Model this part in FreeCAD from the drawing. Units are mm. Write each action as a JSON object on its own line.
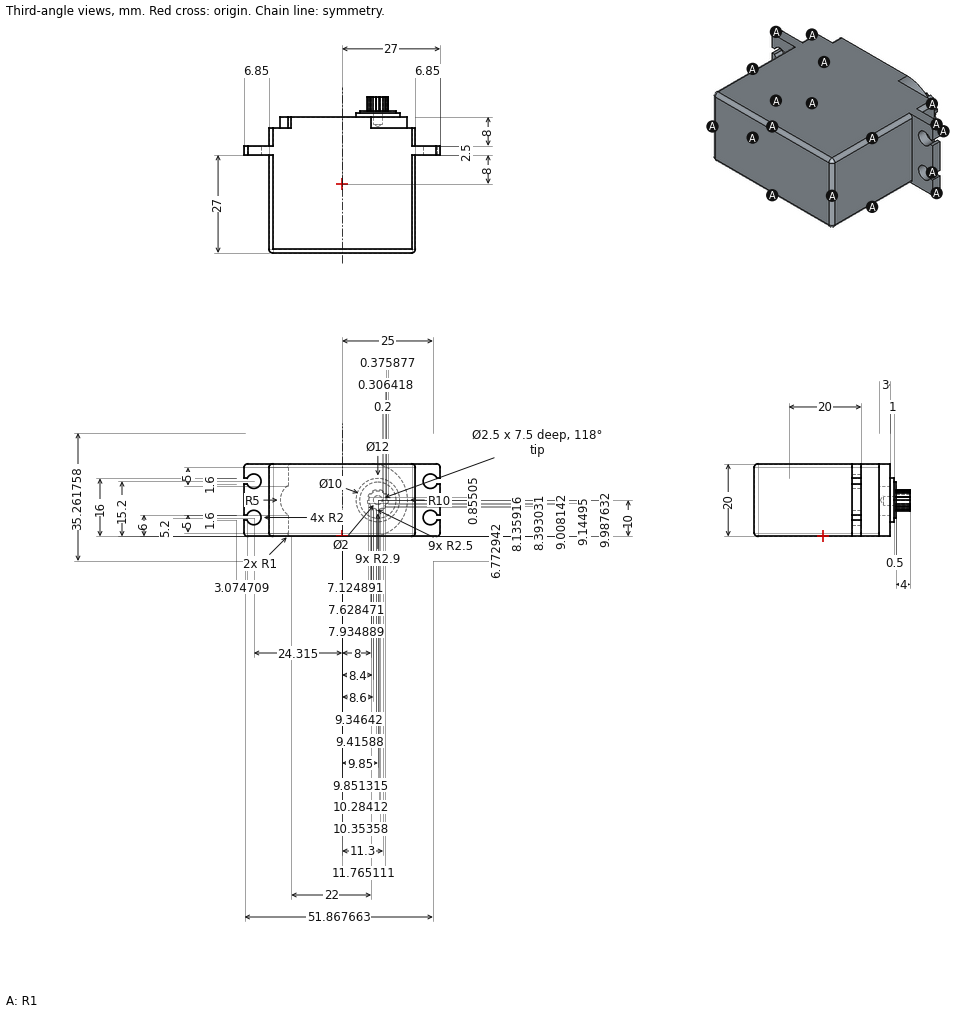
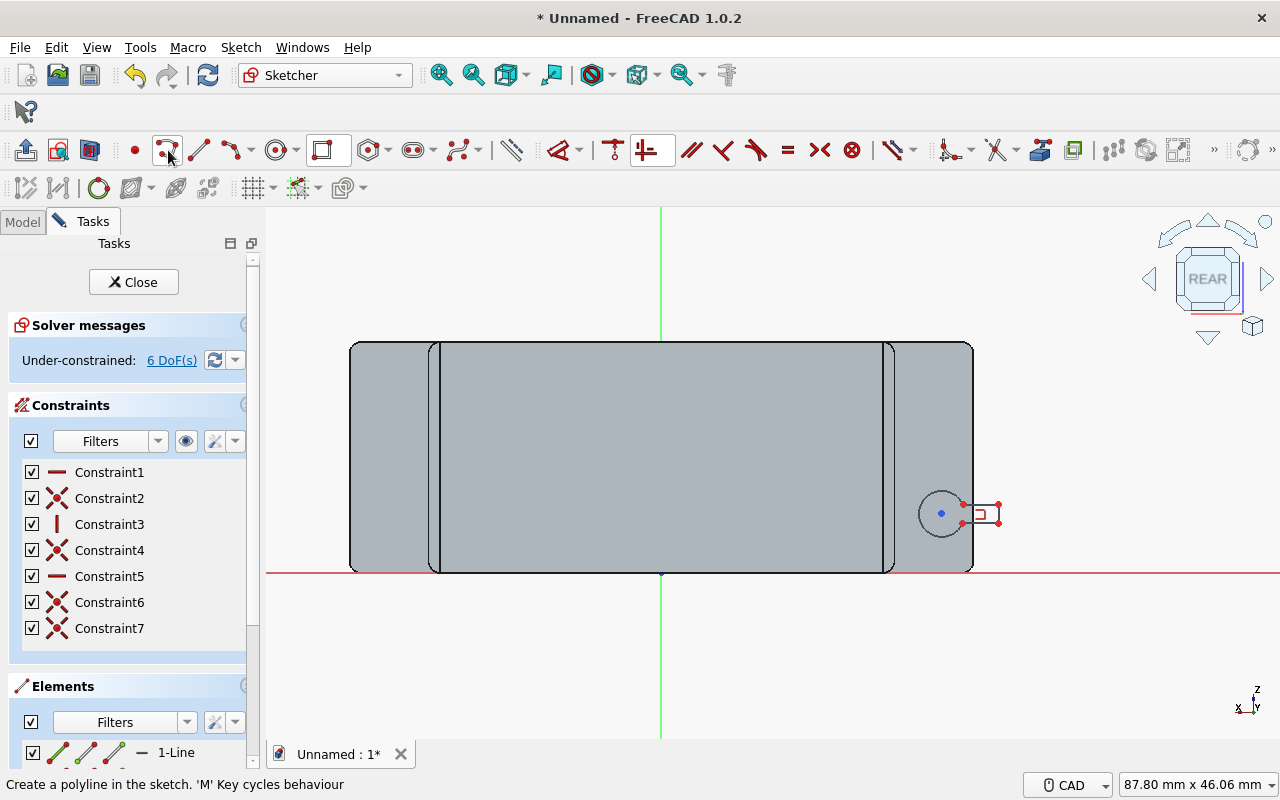
{"action": "left_click", "coordinate": [963, 407]}
{"action": "left_click", "coordinate": [999, 407]}
{"action": "left_click", "coordinate": [999, 388]}
{"action": "left_click", "coordinate": [963, 388]}
{"action": "right_click", "coordinate": [963, 388]}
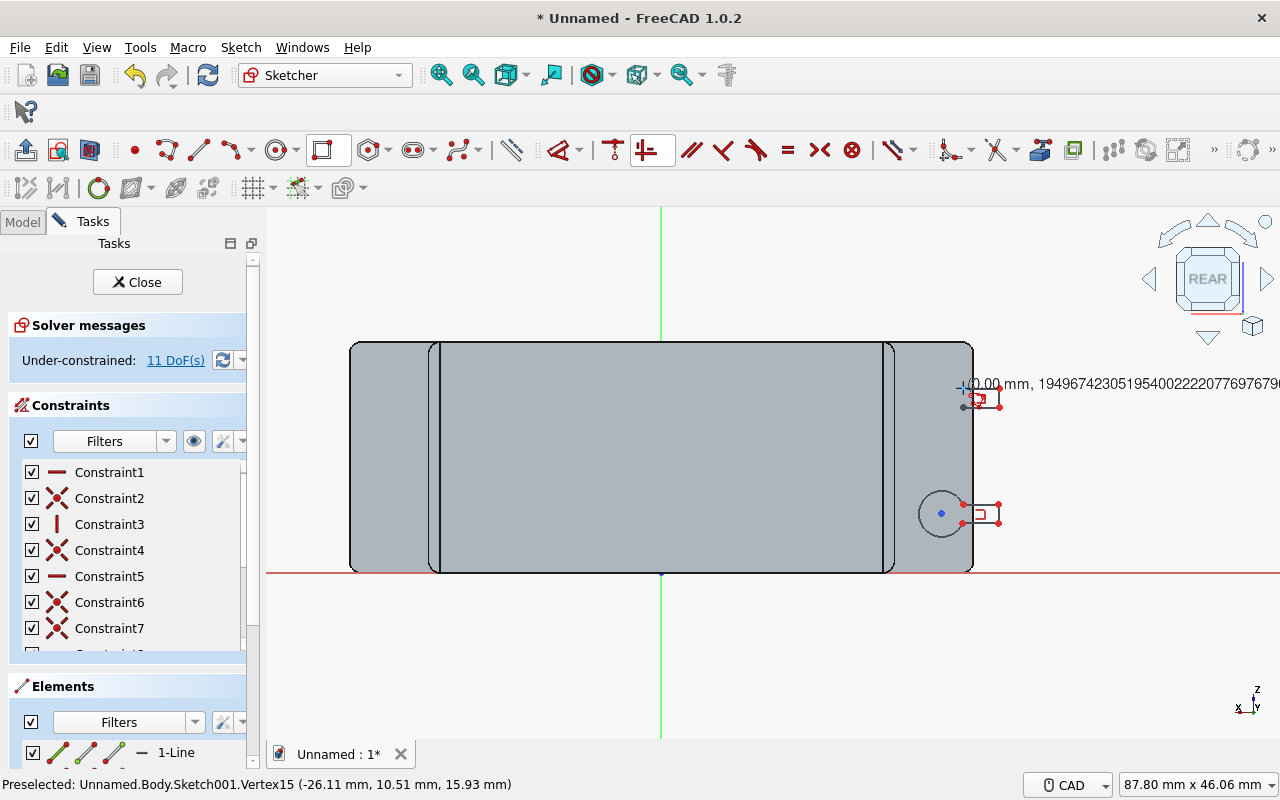
{"action": "left_click", "coordinate": [232, 150]}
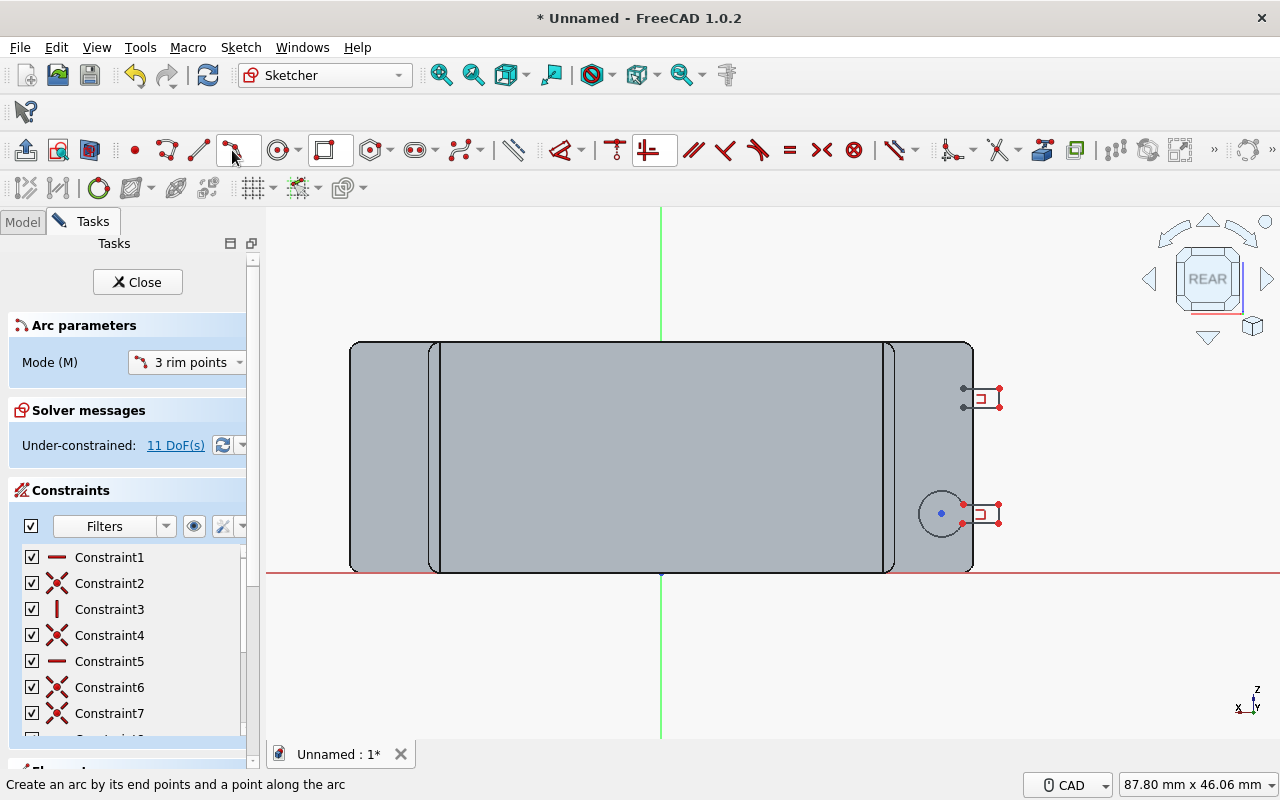
{"action": "left_click", "coordinate": [963, 389]}
{"action": "left_click", "coordinate": [963, 408]}
{"action": "left_click", "coordinate": [919, 397]}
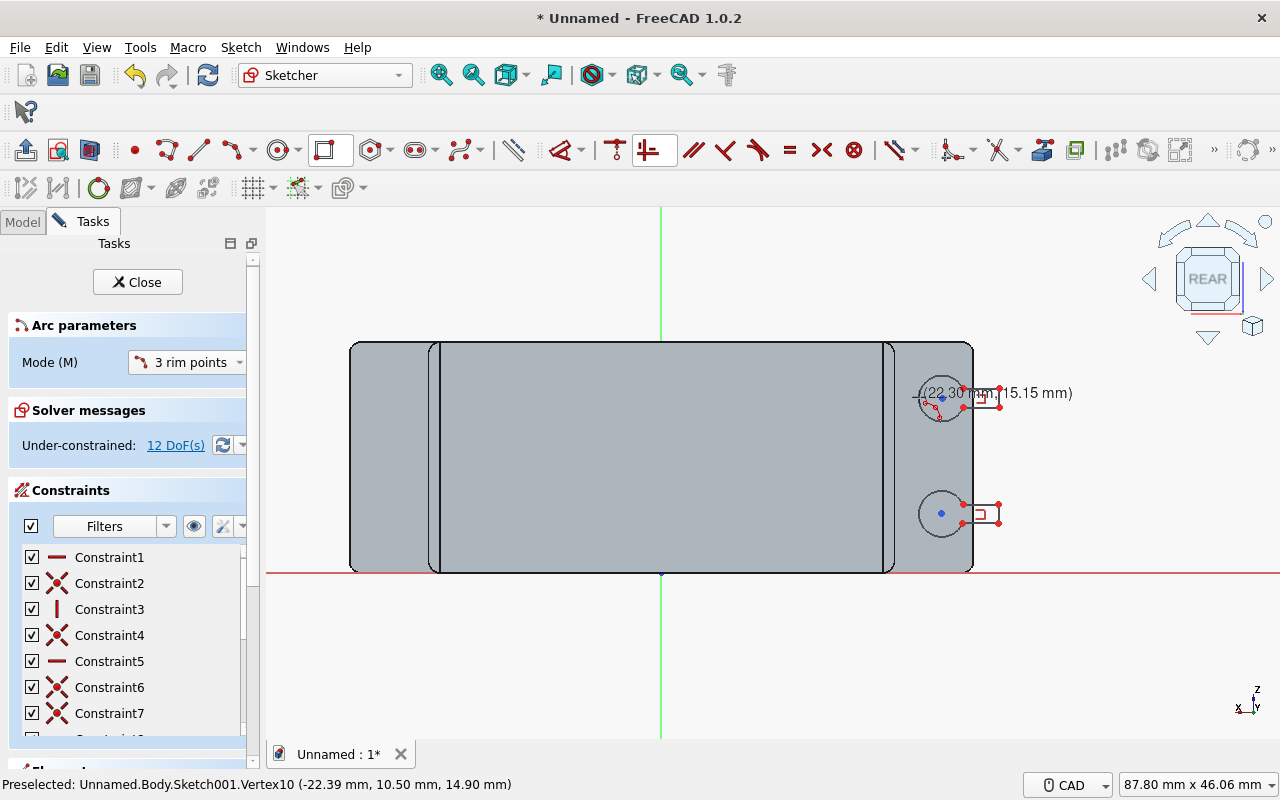
{"action": "left_click", "coordinate": [168, 150]}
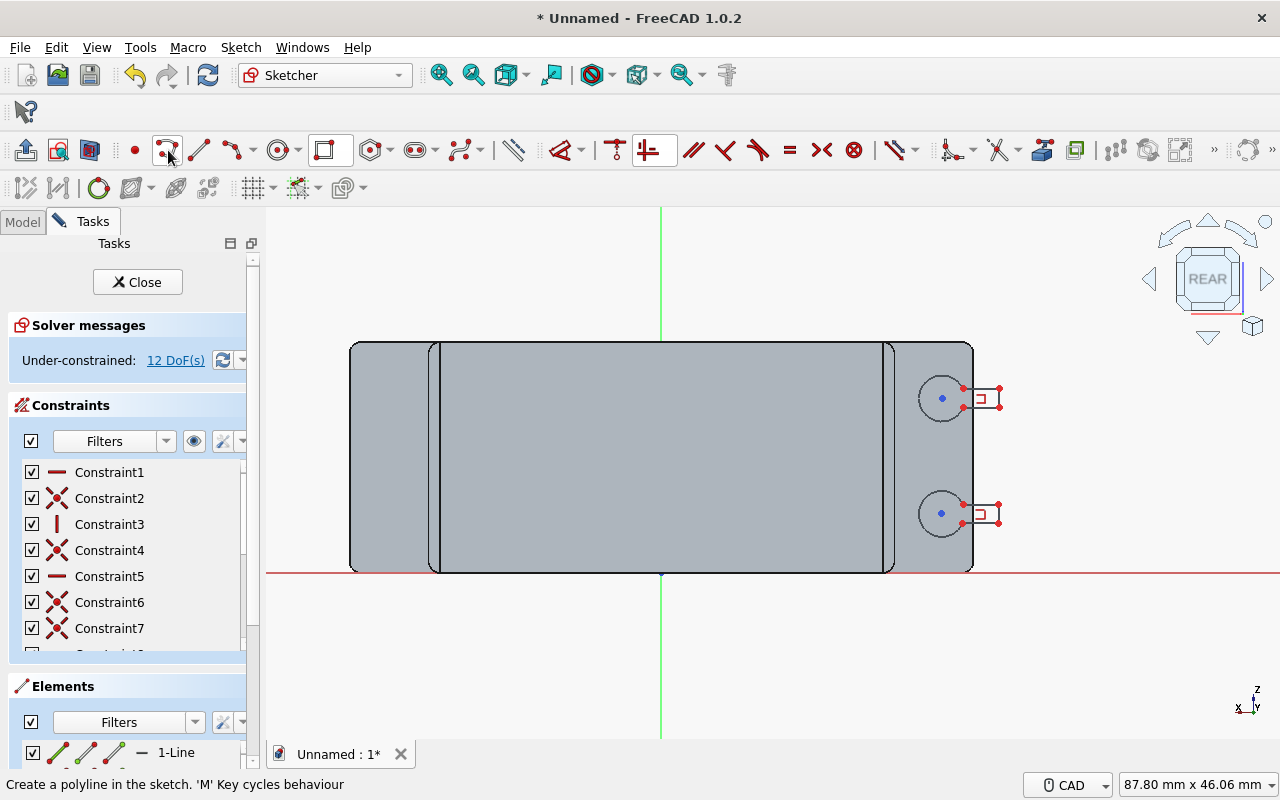
{"action": "left_click", "coordinate": [360, 388]}
{"action": "left_click", "coordinate": [324, 388]}
{"action": "left_click", "coordinate": [324, 407]}
{"action": "left_click", "coordinate": [360, 407]}
{"action": "right_click", "coordinate": [360, 407]}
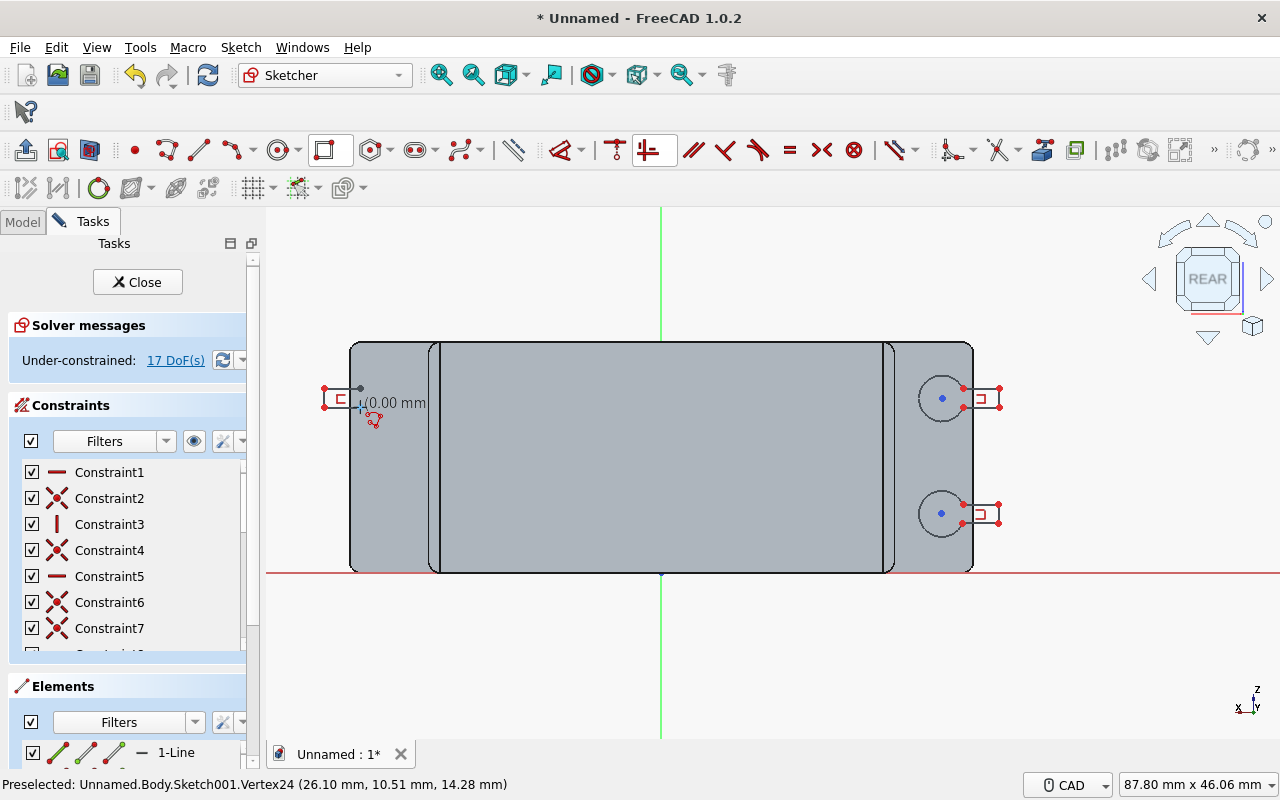
{"action": "left_click", "coordinate": [232, 150]}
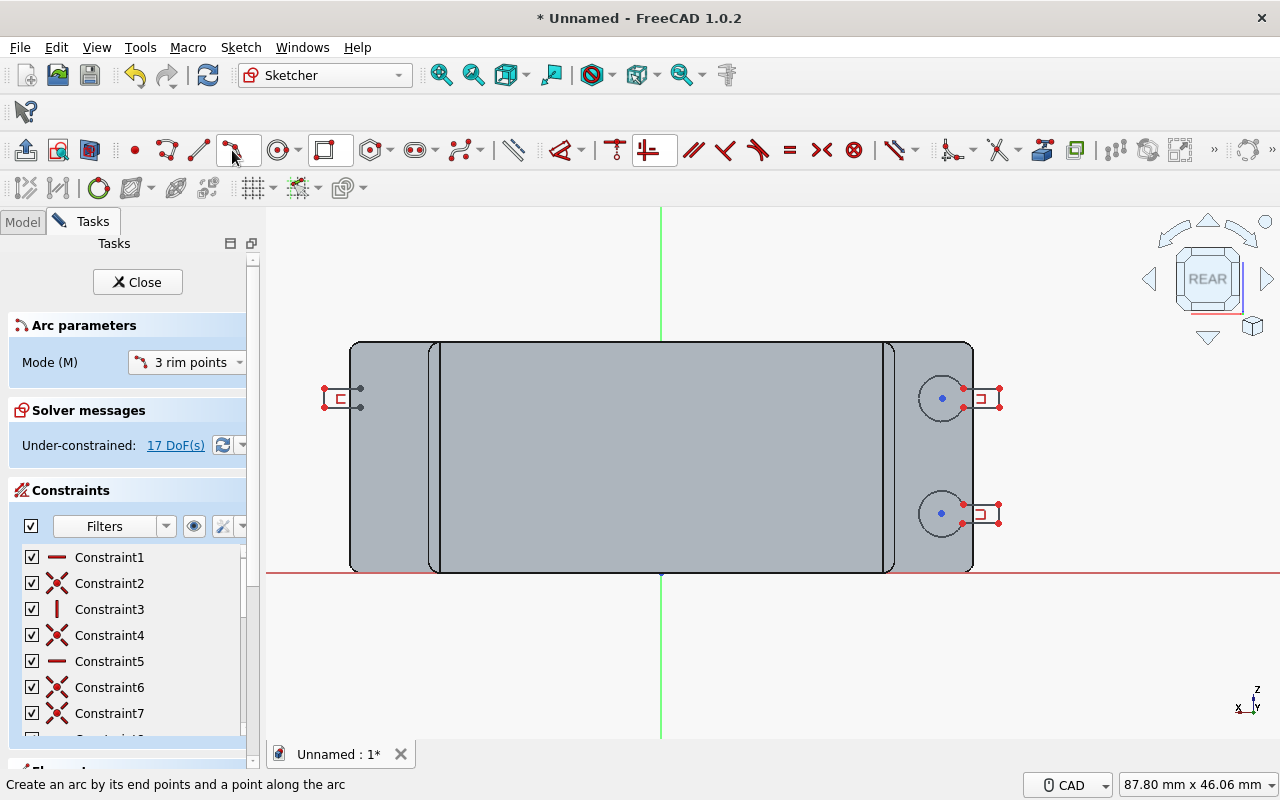
{"action": "left_click", "coordinate": [360, 408]}
{"action": "left_click", "coordinate": [360, 389]}
{"action": "left_click", "coordinate": [404, 397]}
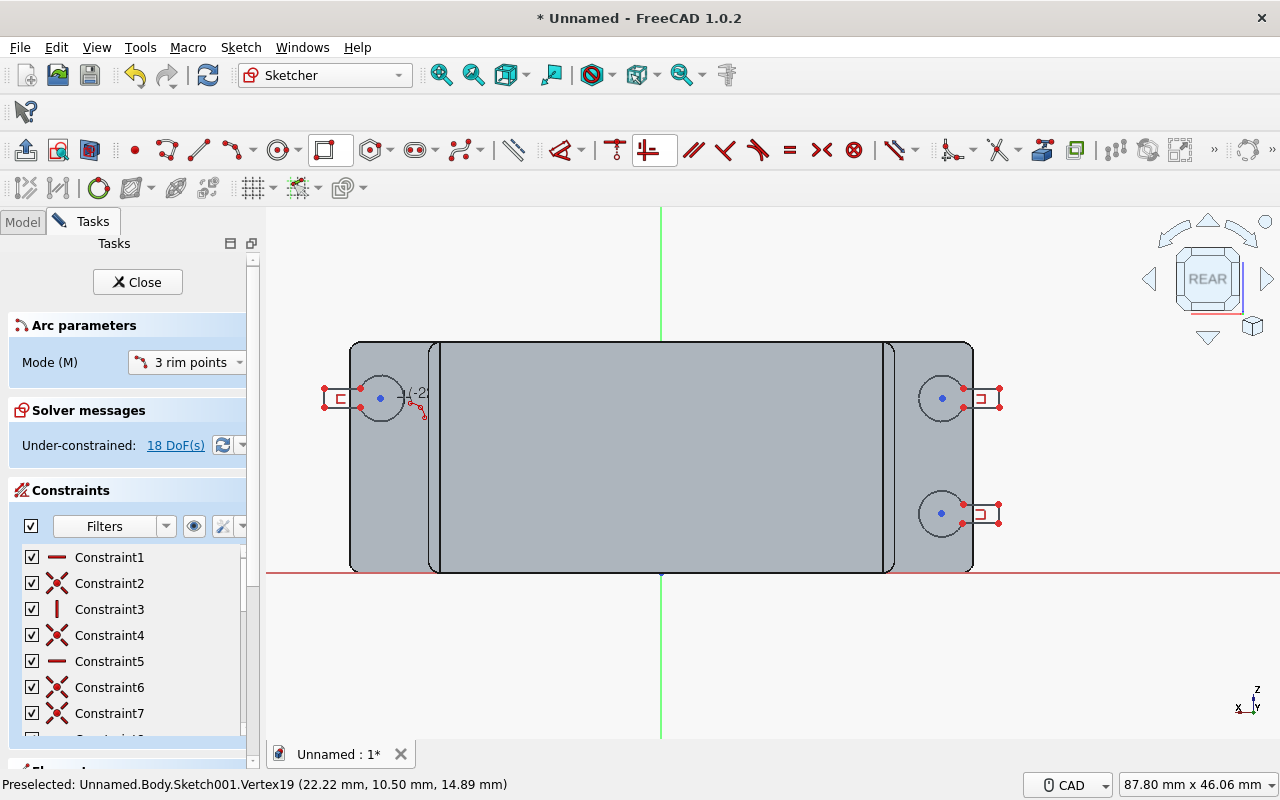
{"action": "left_click", "coordinate": [168, 150]}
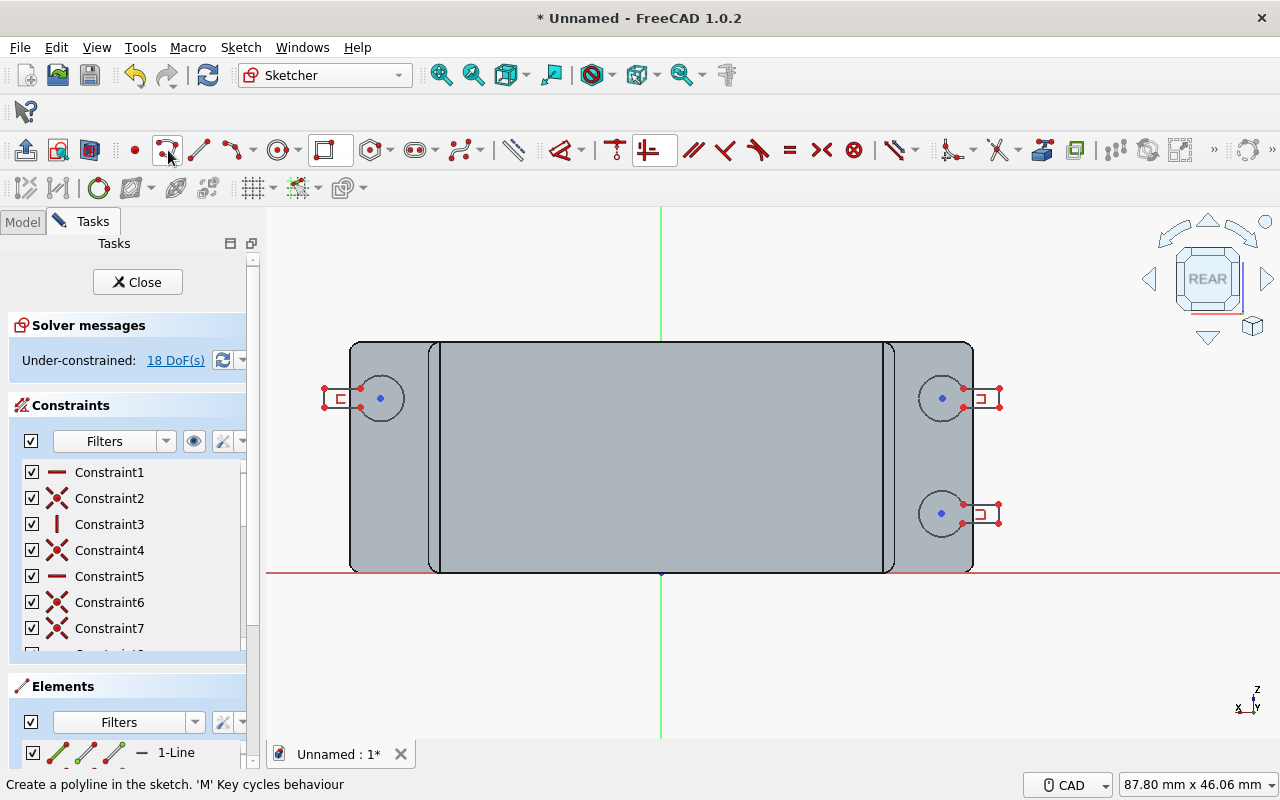
{"action": "left_click", "coordinate": [360, 504]}
{"action": "left_click", "coordinate": [324, 504]}
{"action": "left_click", "coordinate": [324, 522]}
{"action": "left_click", "coordinate": [360, 522]}
{"action": "right_click", "coordinate": [360, 522]}